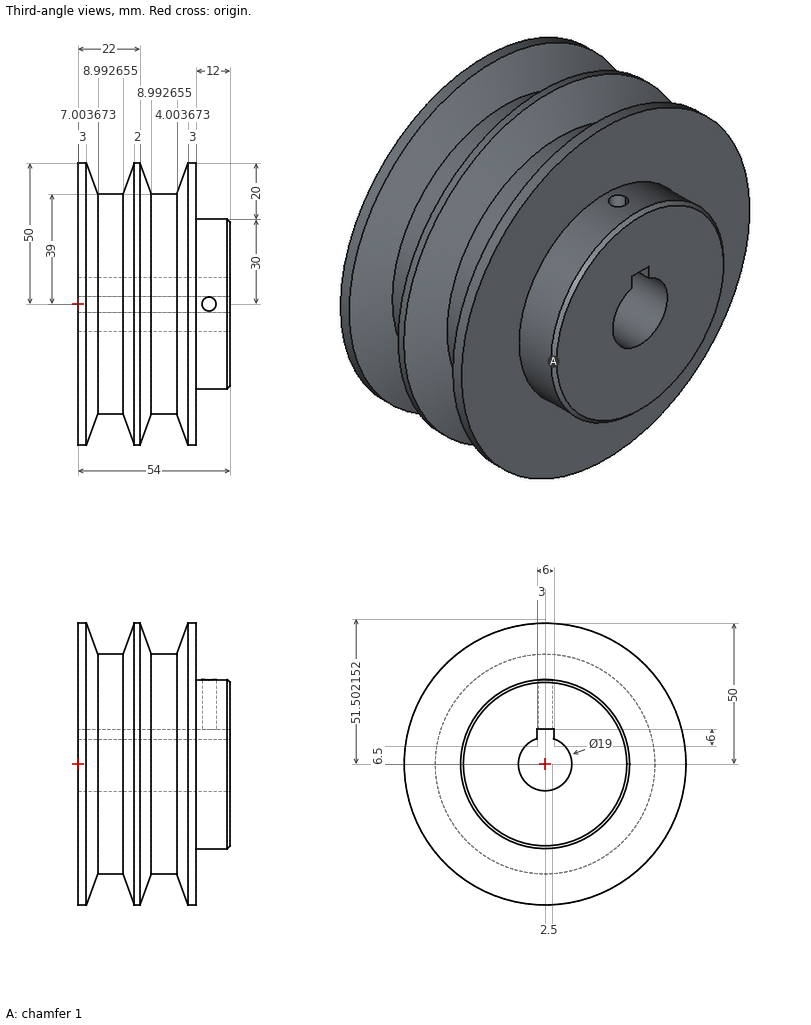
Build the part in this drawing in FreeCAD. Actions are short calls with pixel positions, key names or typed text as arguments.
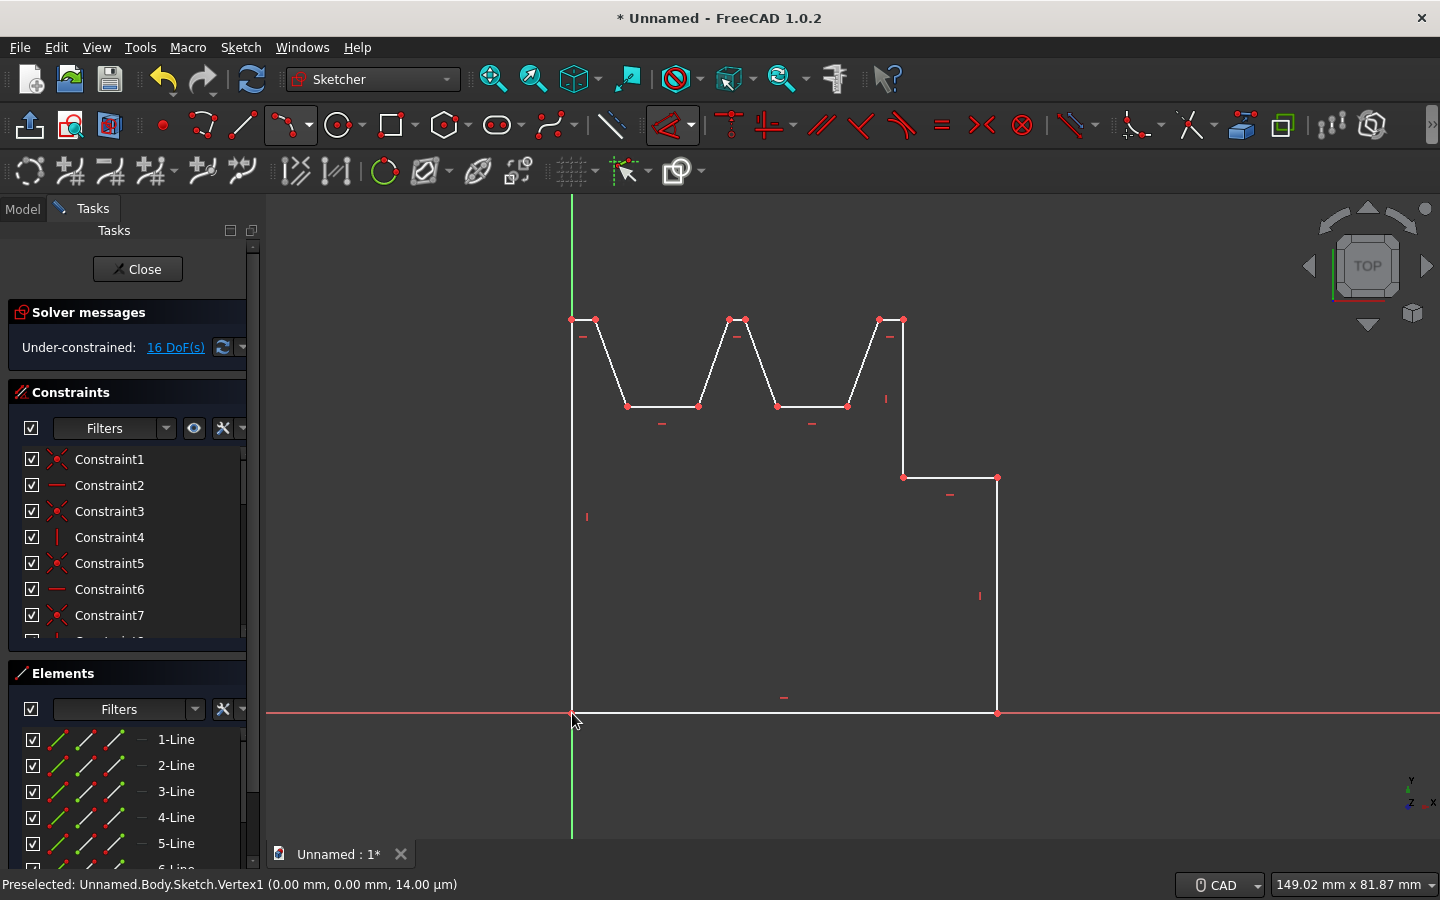
click(666, 126)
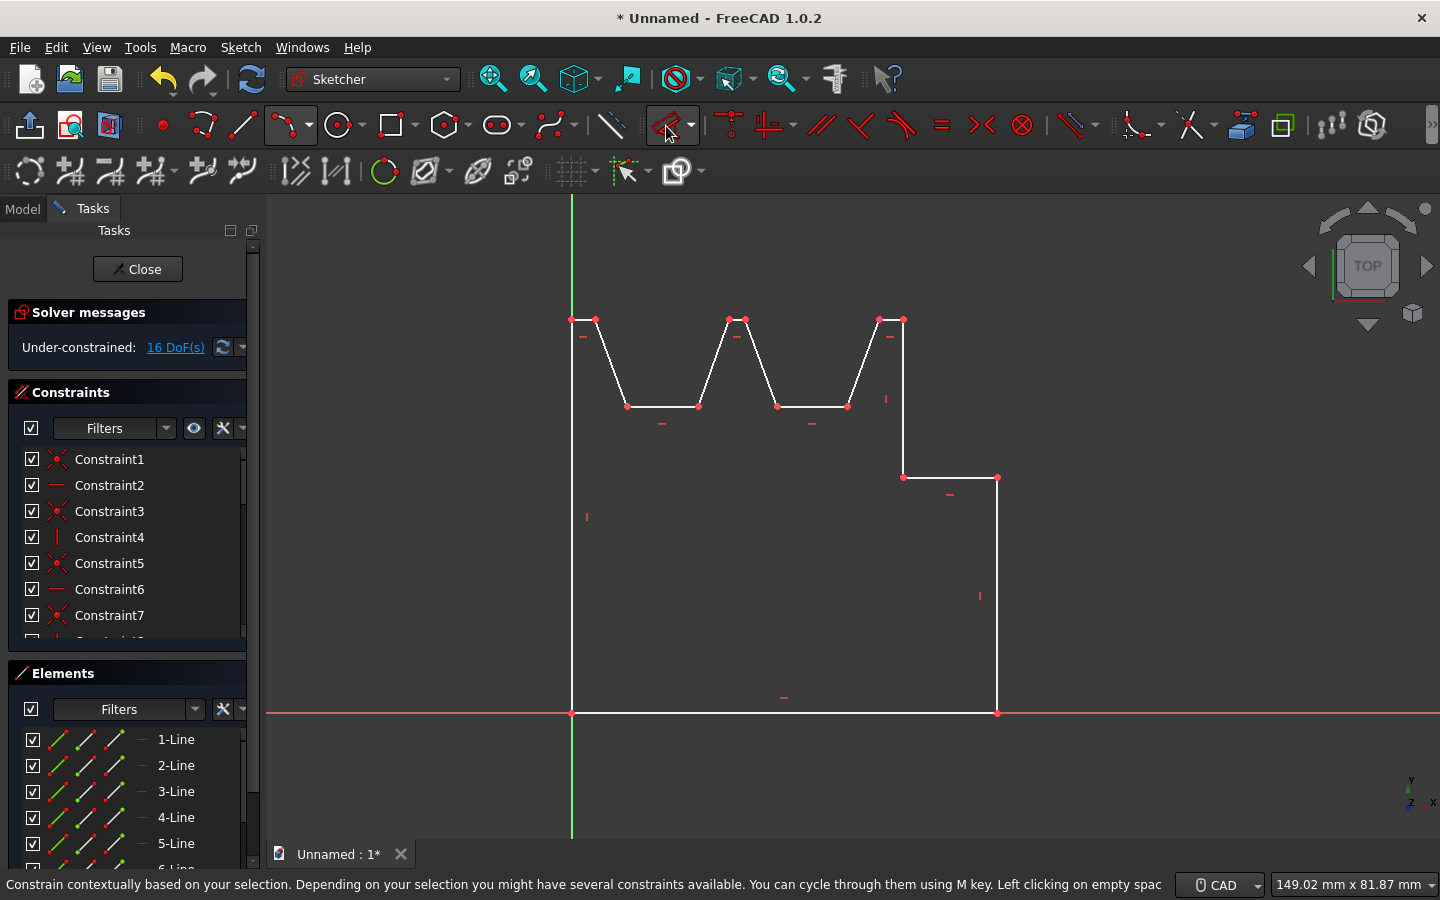
scroll(893, 320, up, 3)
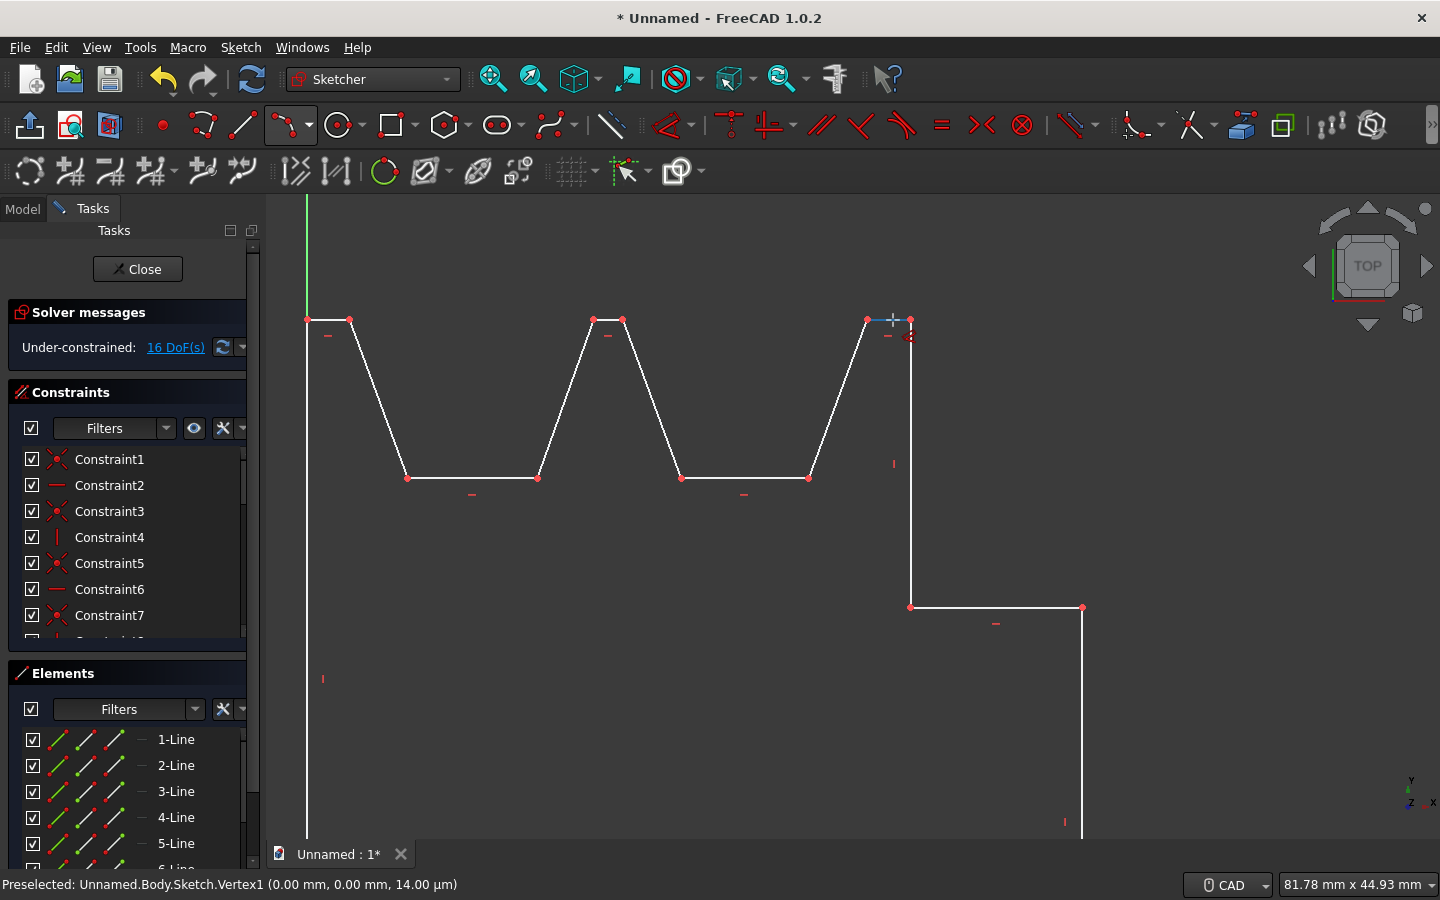
click(893, 320)
click(889, 286)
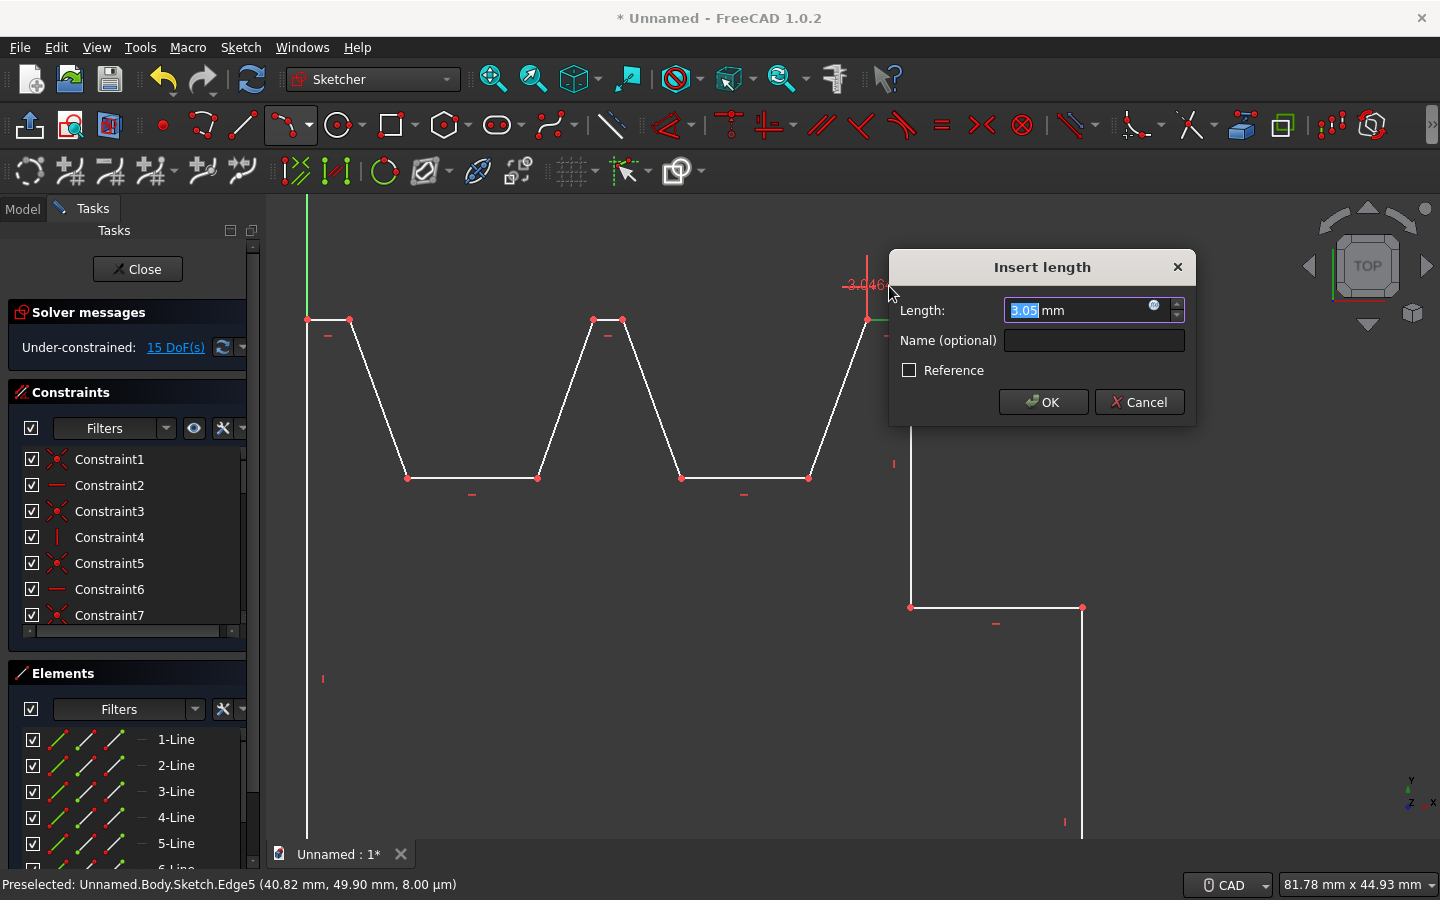
text(3)
key(Return)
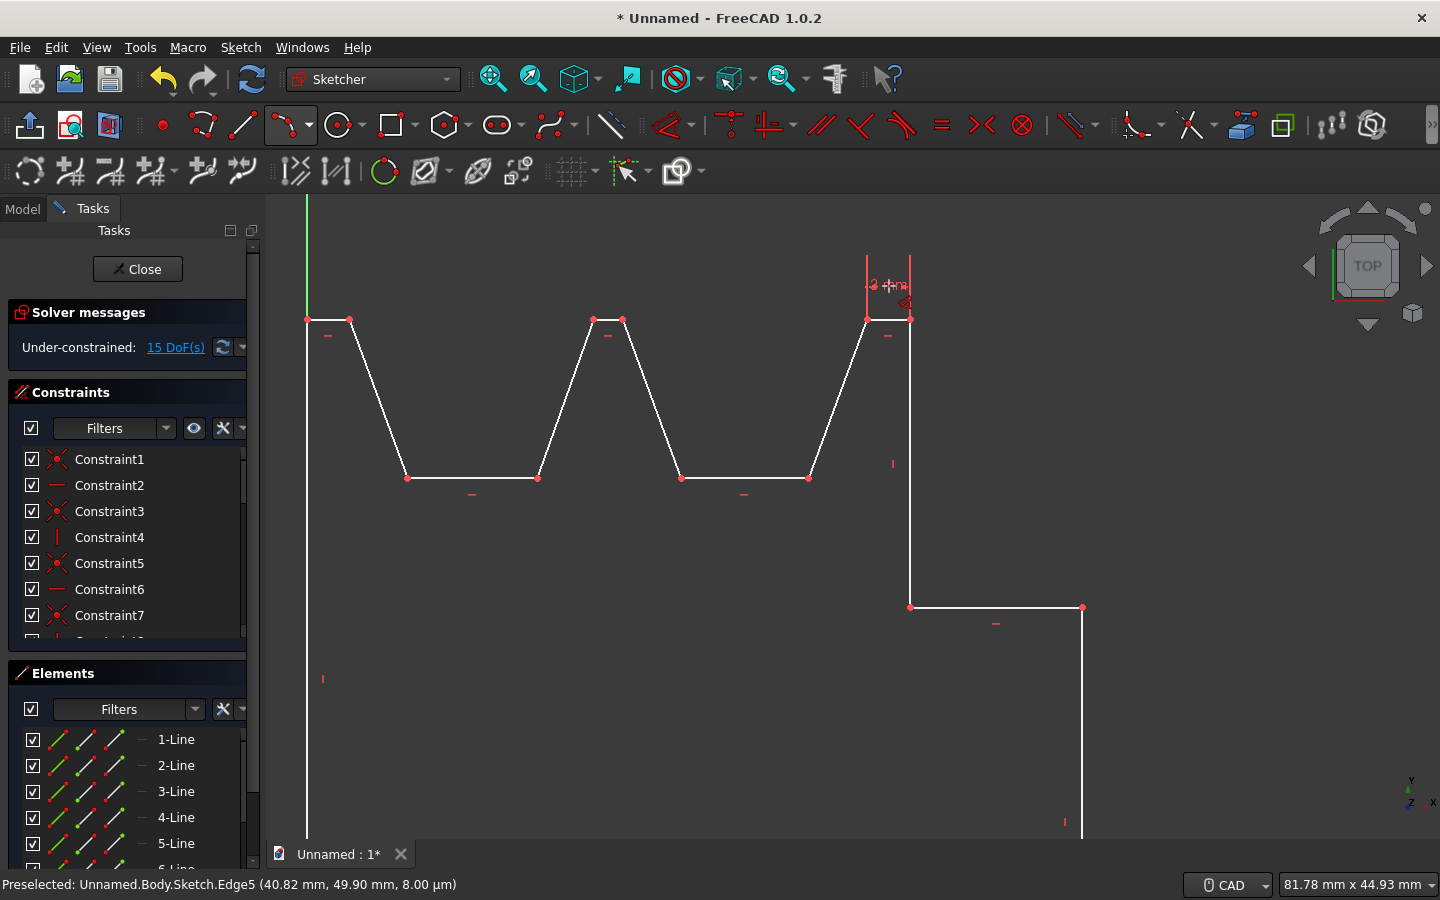
scroll(611, 320, up, 2)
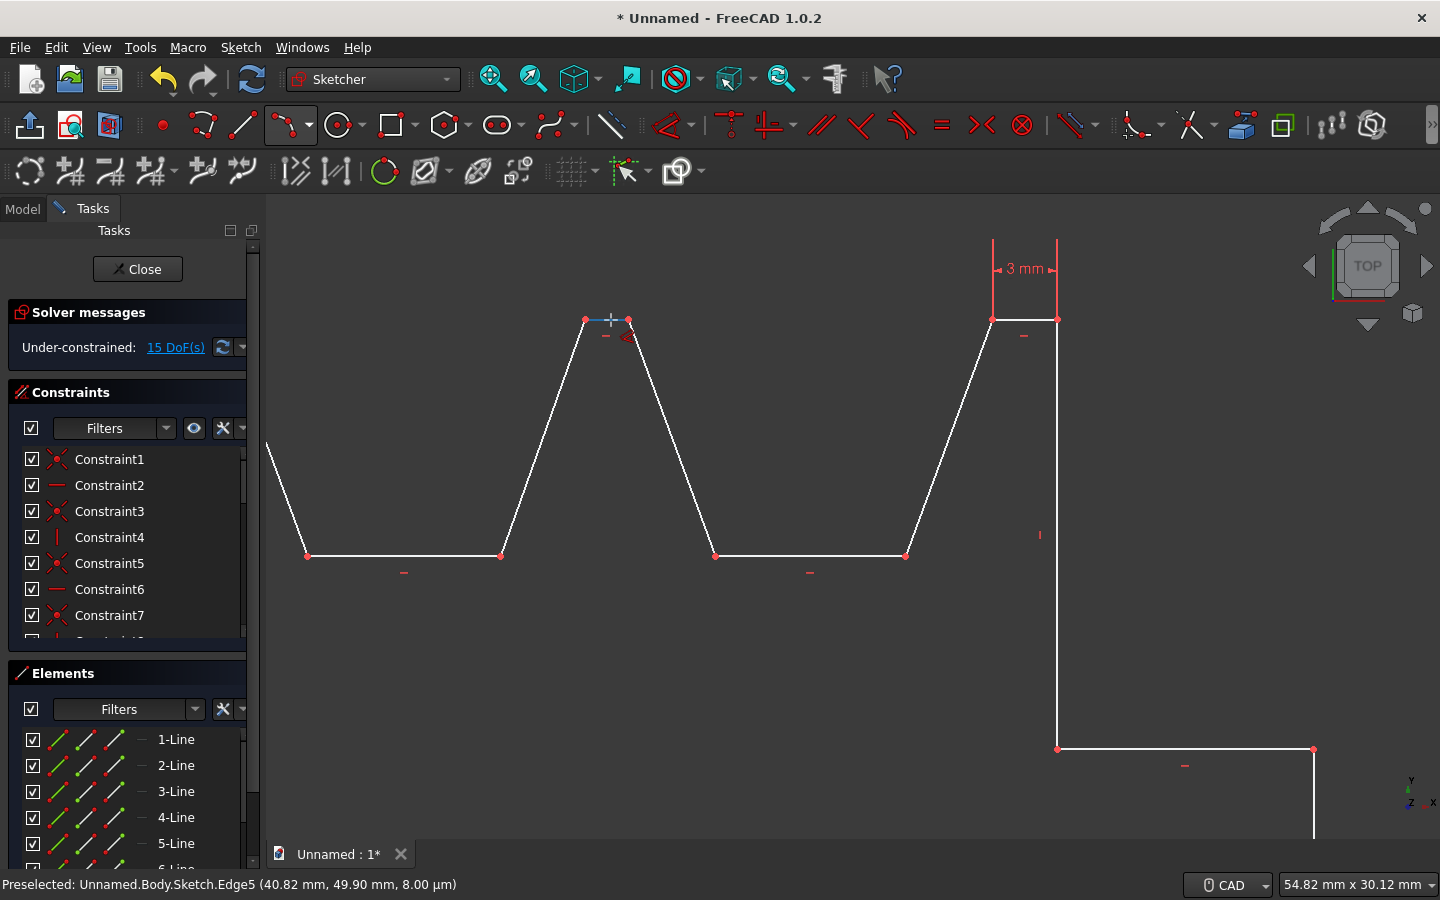
click(611, 320)
click(607, 286)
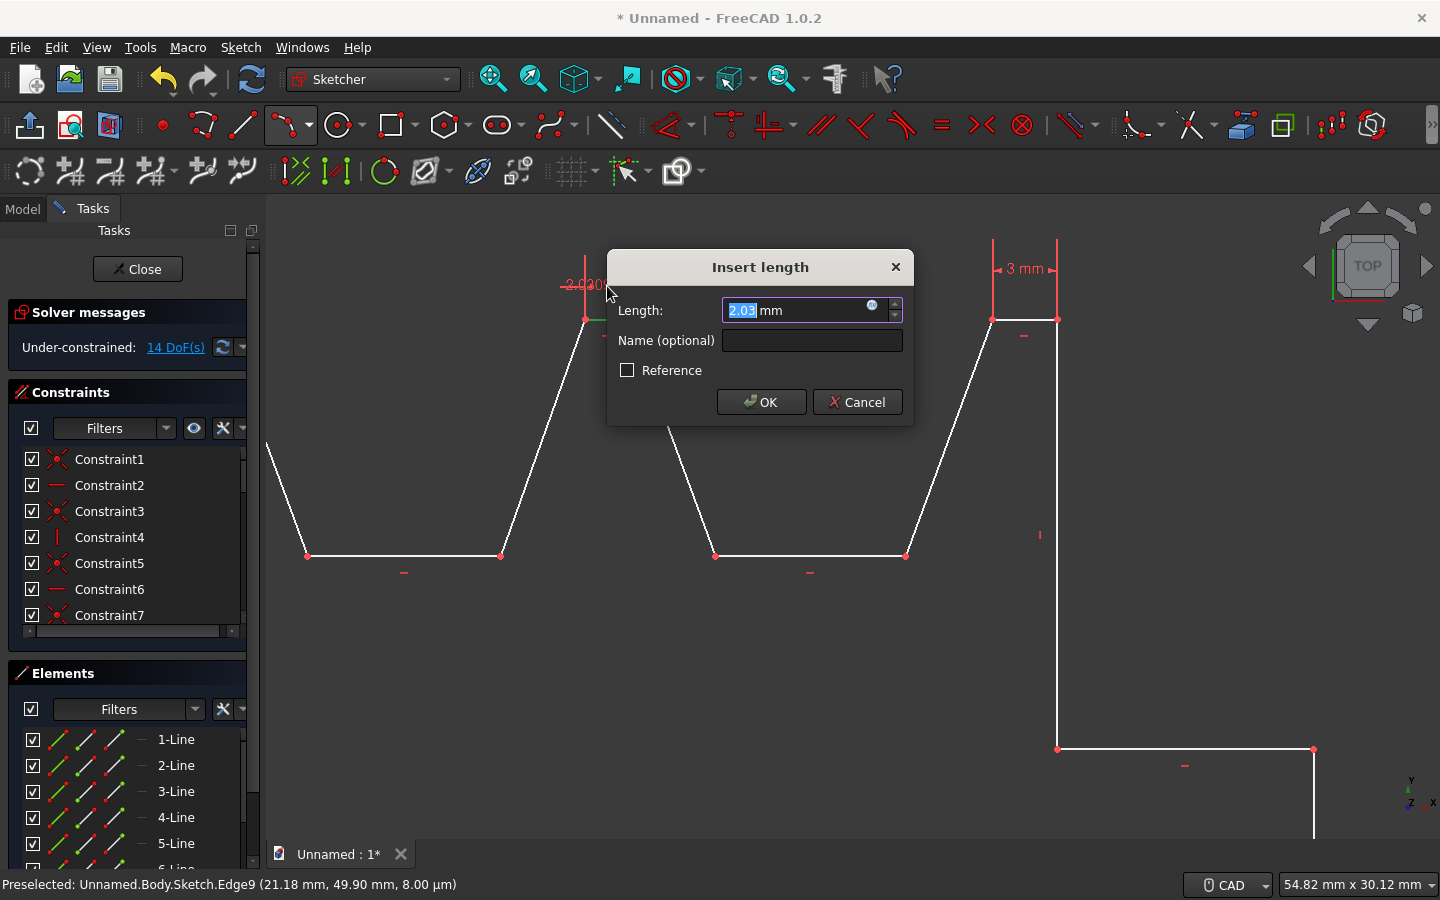
text(2)
key(Return)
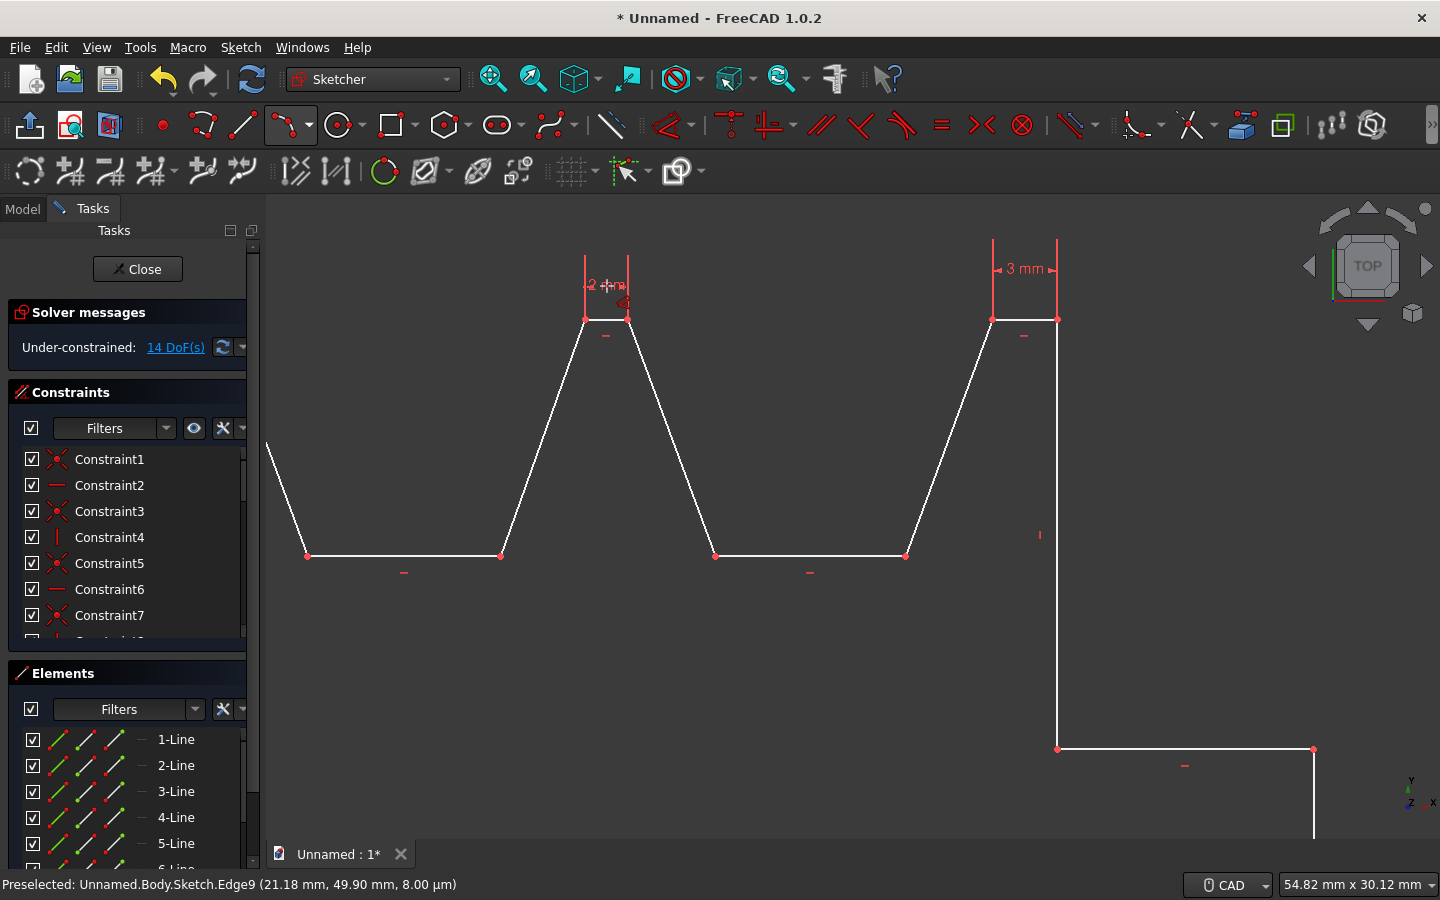
scroll(813, 321, down, 5)